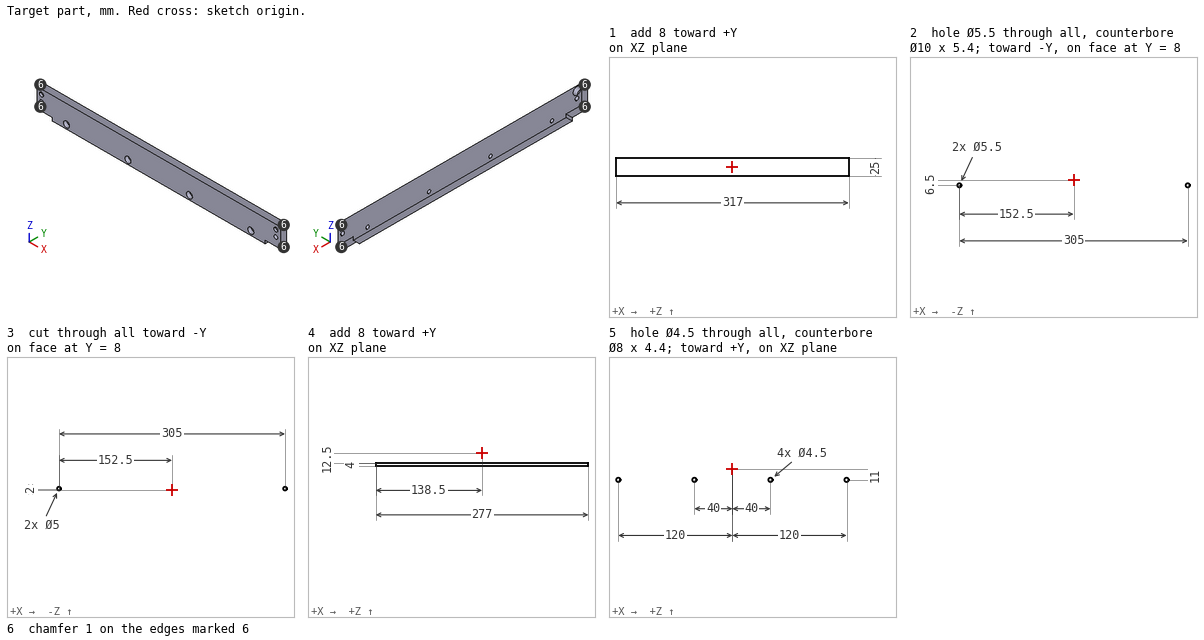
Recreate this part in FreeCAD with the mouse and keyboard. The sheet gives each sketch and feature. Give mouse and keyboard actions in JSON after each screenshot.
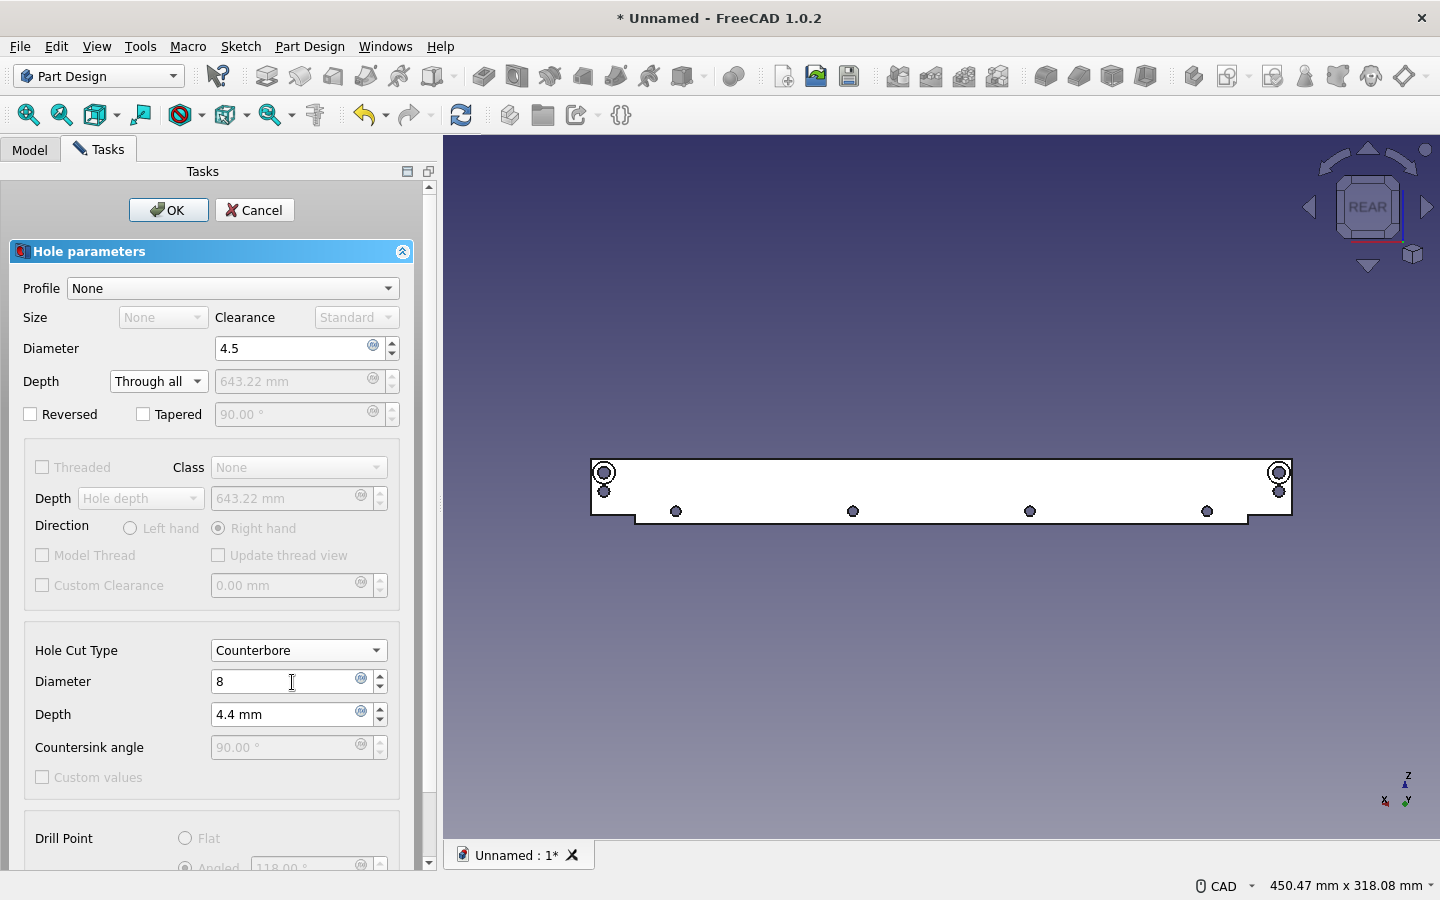
{"action": "left_click", "coordinate": [169, 210]}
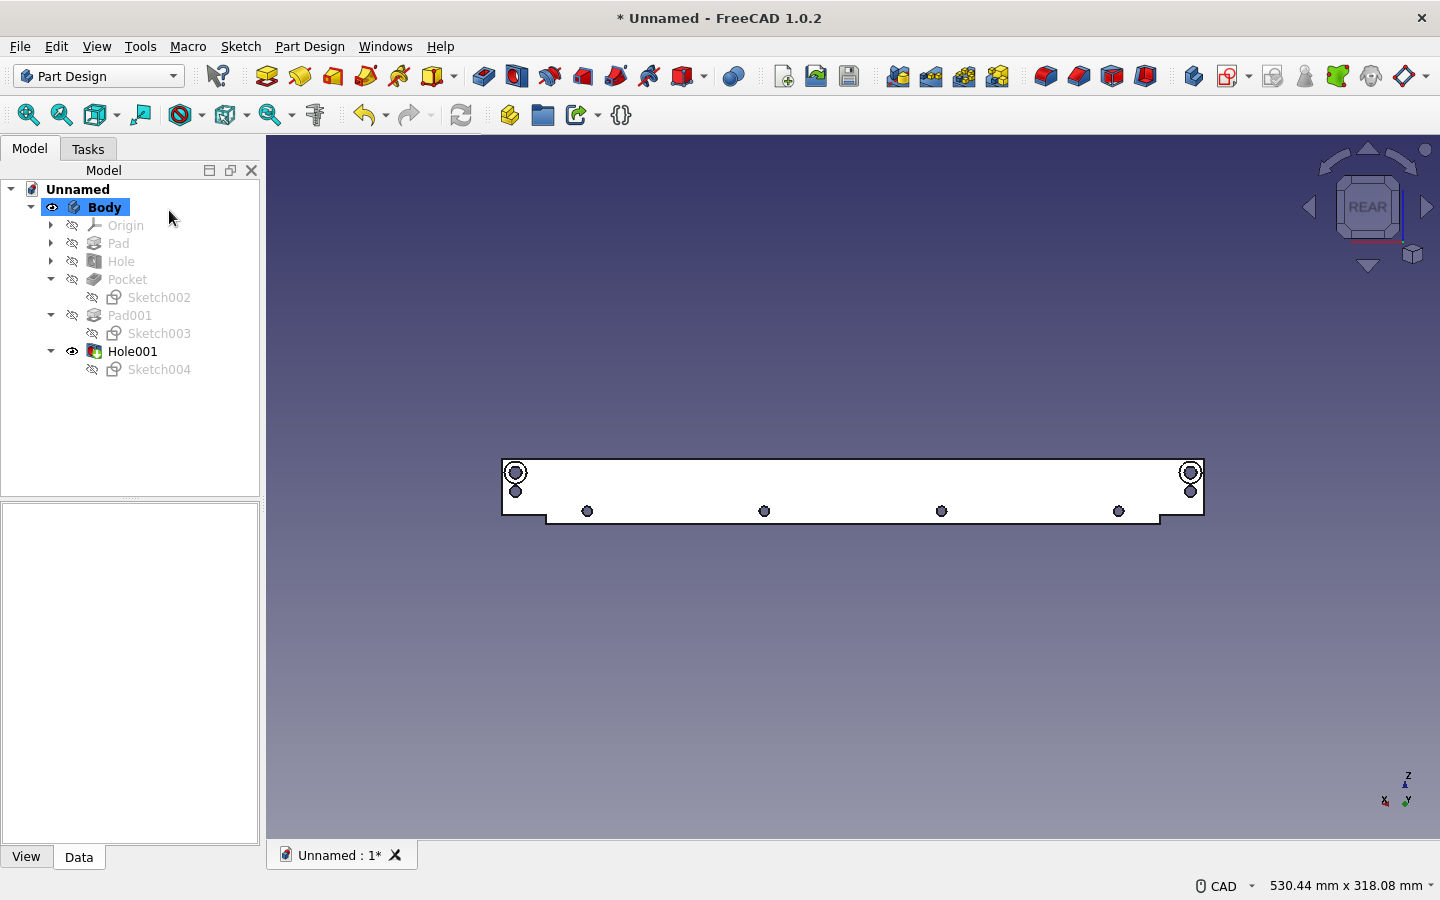
{"action": "scroll", "coordinate": [1204, 514], "scroll_direction": "up", "scroll_amount": 5}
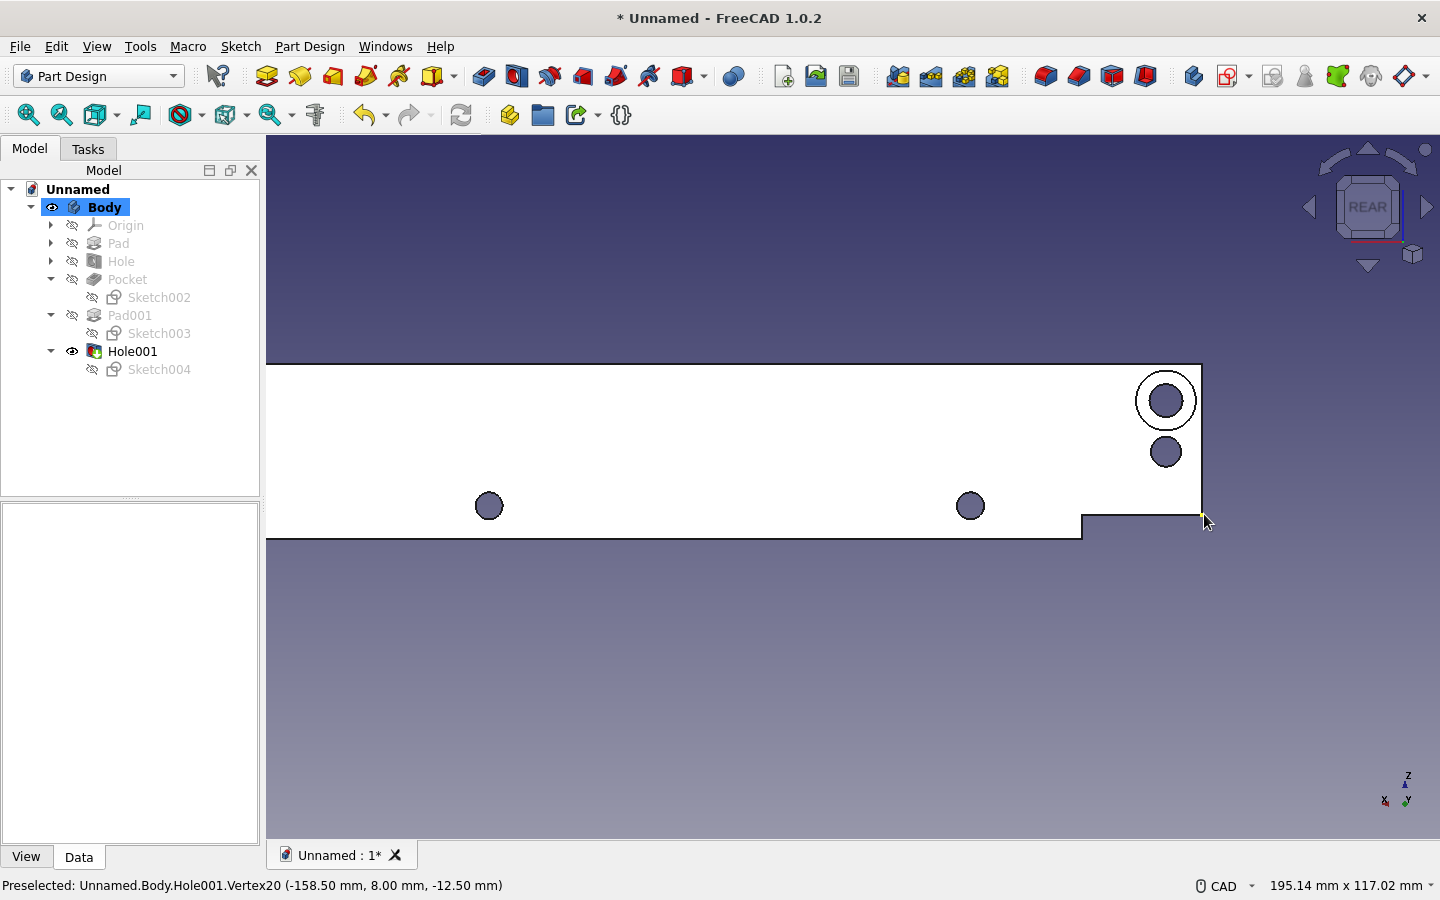
{"action": "left_click", "coordinate": [29, 116]}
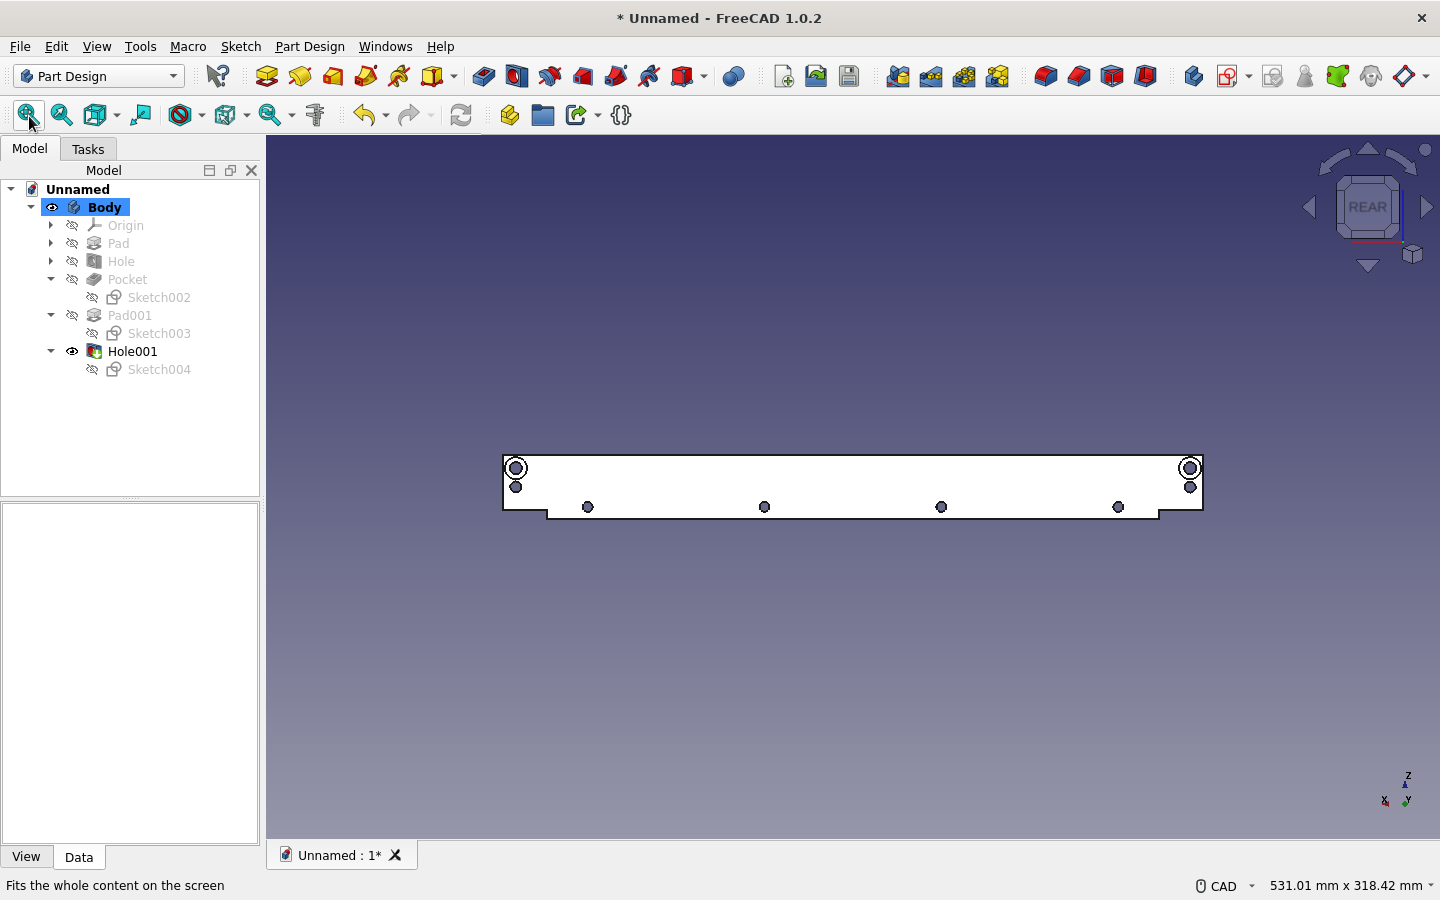
{"action": "key", "text": "0"}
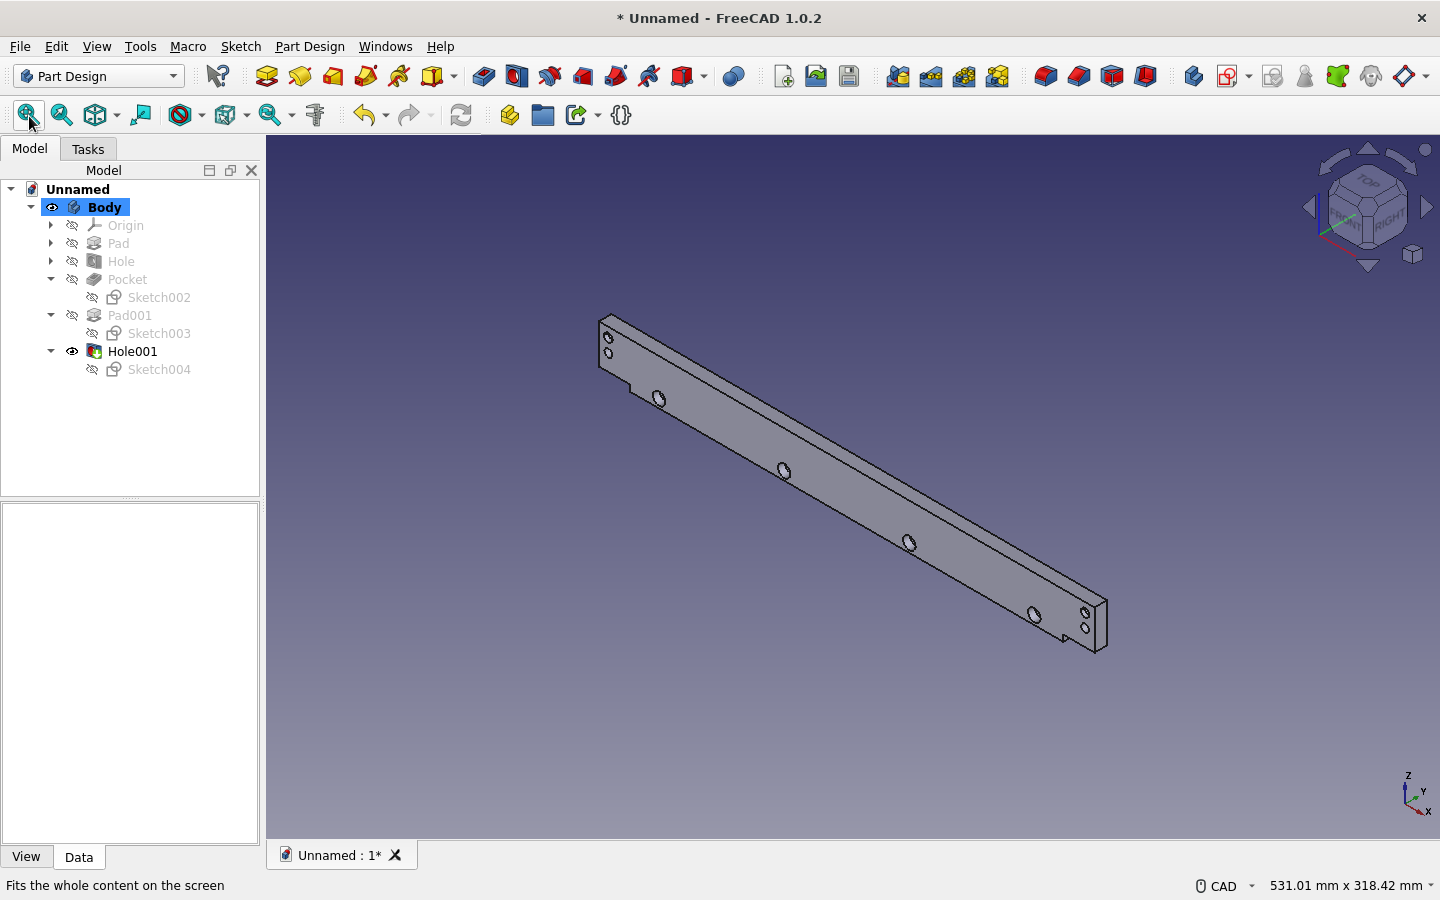
{"action": "left_click", "coordinate": [1101, 603]}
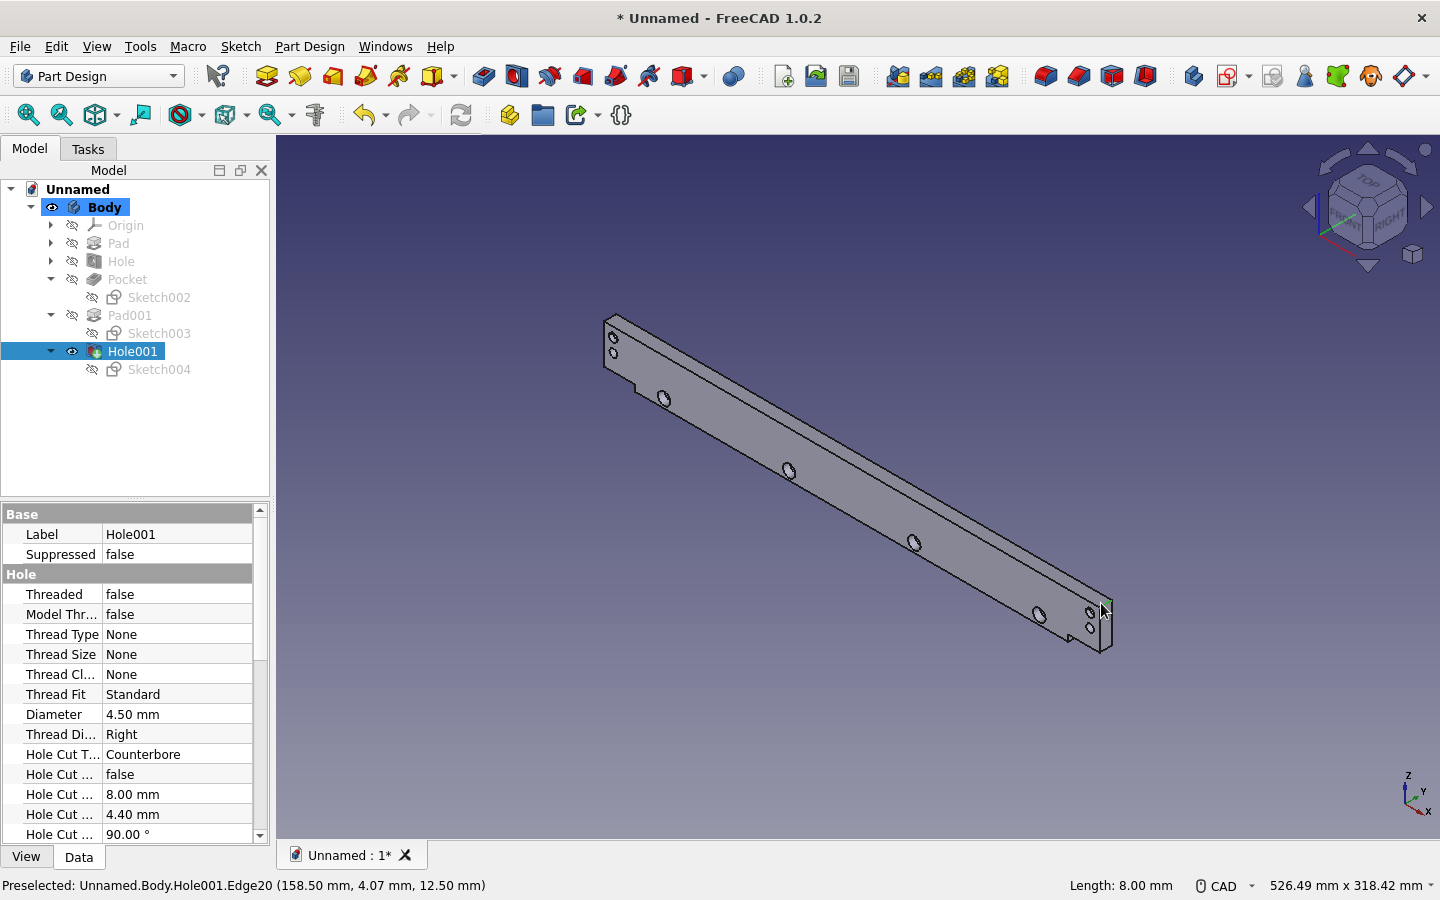
{"action": "scroll", "coordinate": [610, 362], "scroll_direction": "up", "scroll_amount": 5}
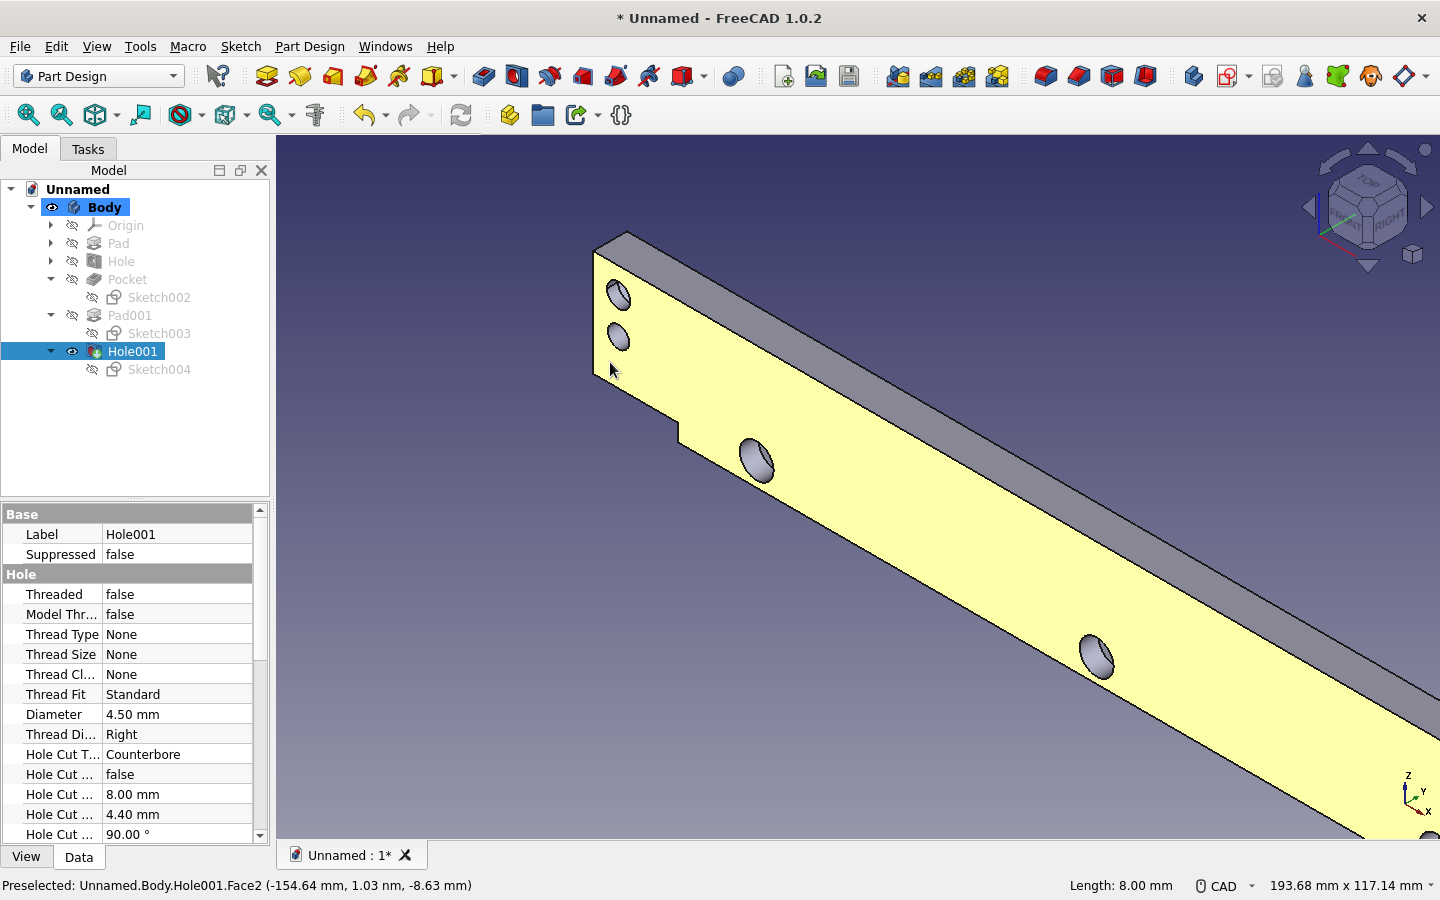
{"action": "left_click", "coordinate": [29, 116]}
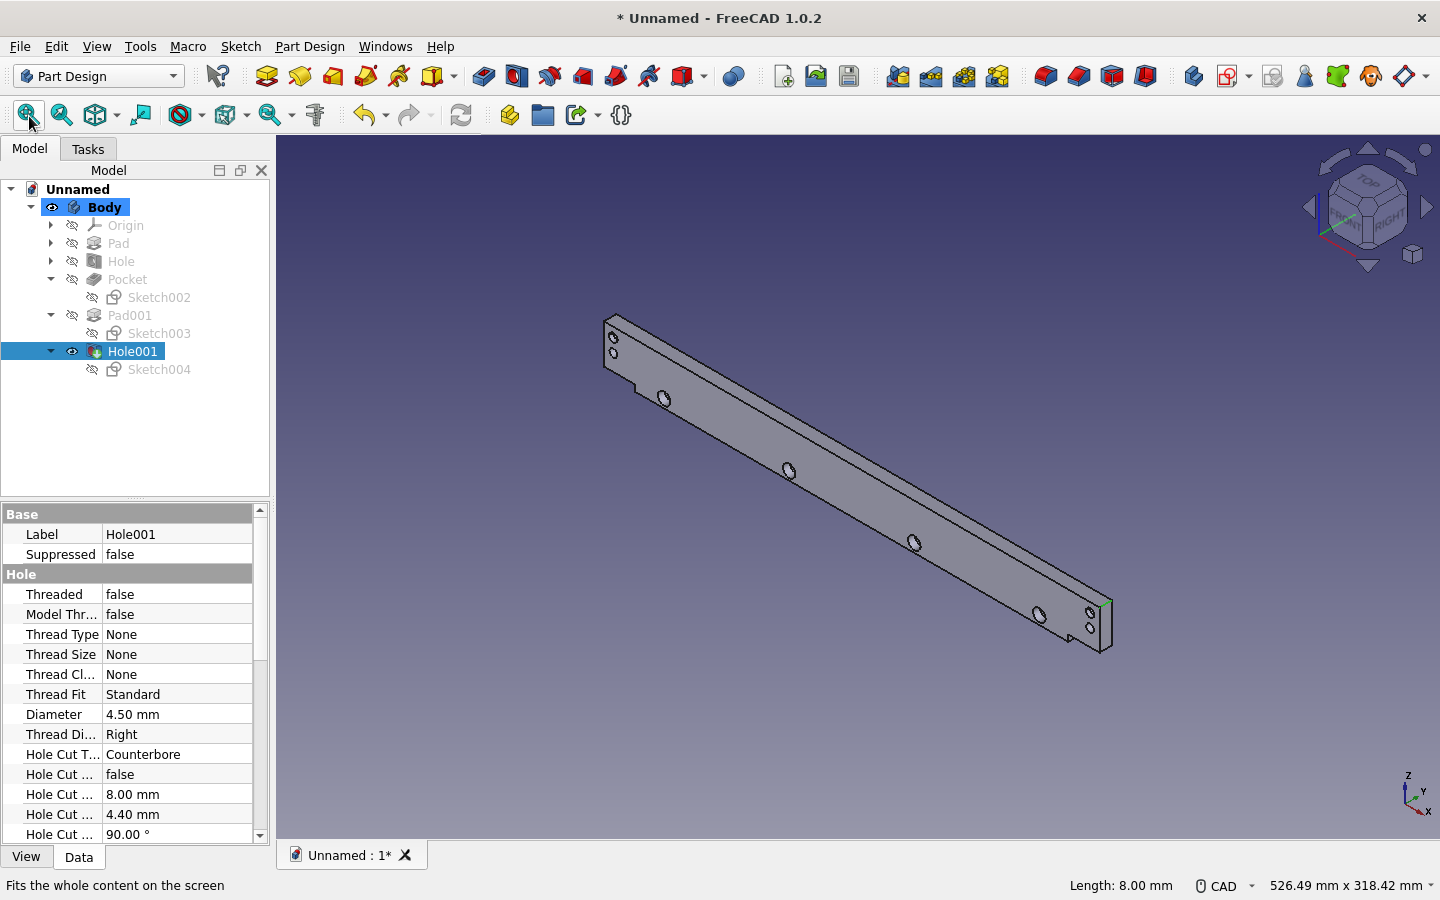
{"action": "key", "text": "2"}